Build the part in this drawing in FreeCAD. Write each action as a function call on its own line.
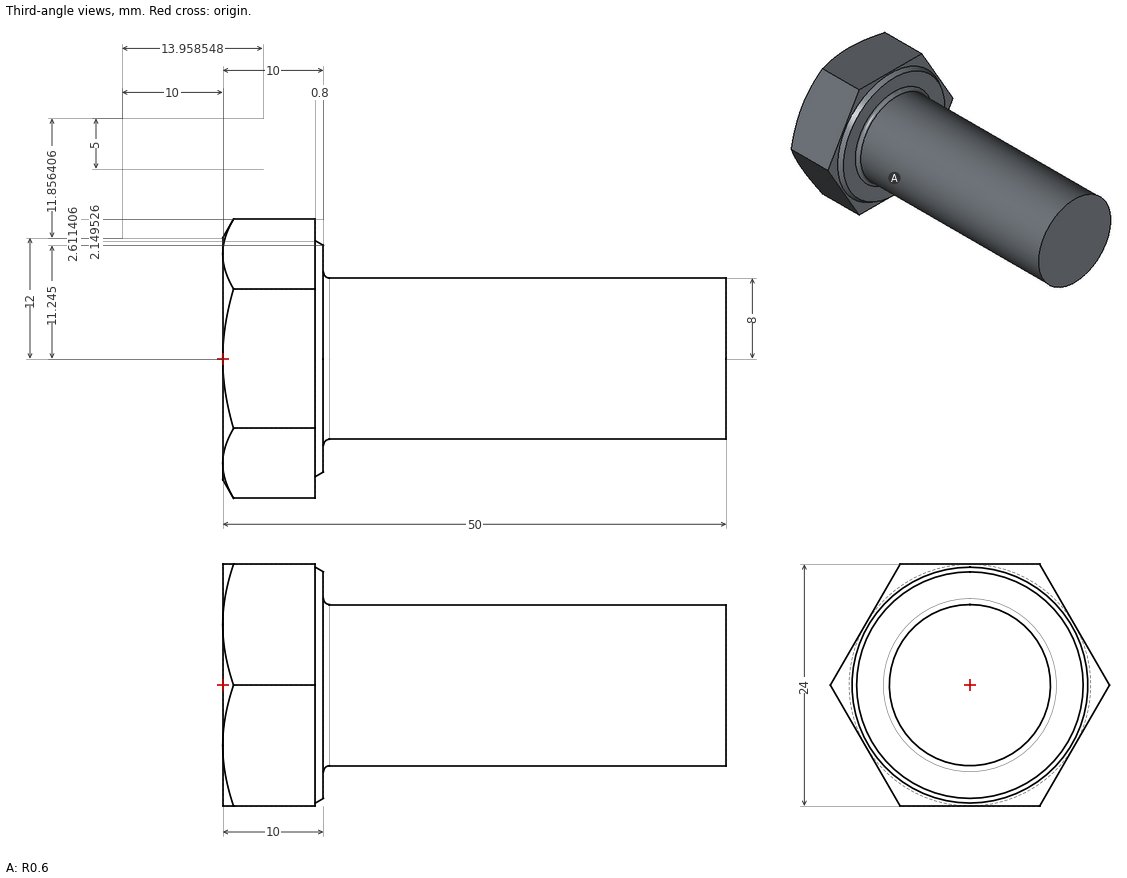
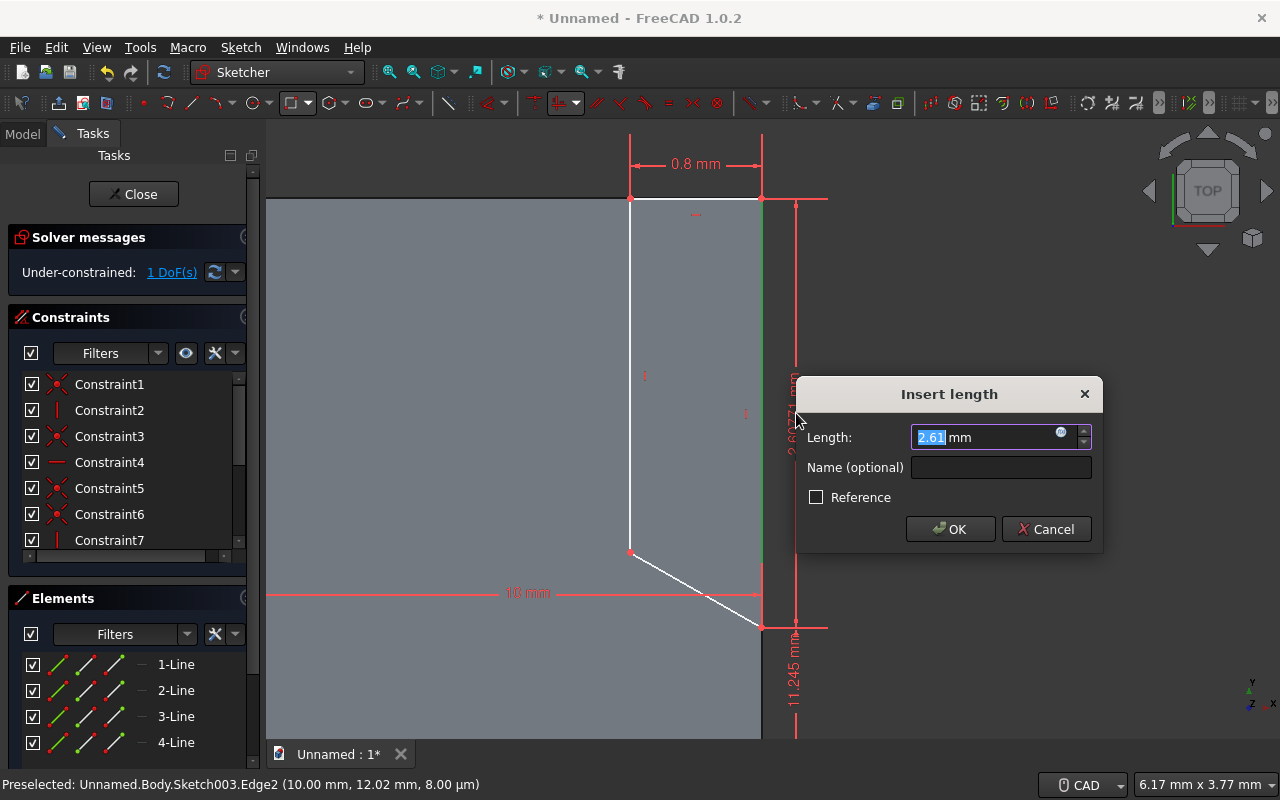
text(2.611406)
key(Return)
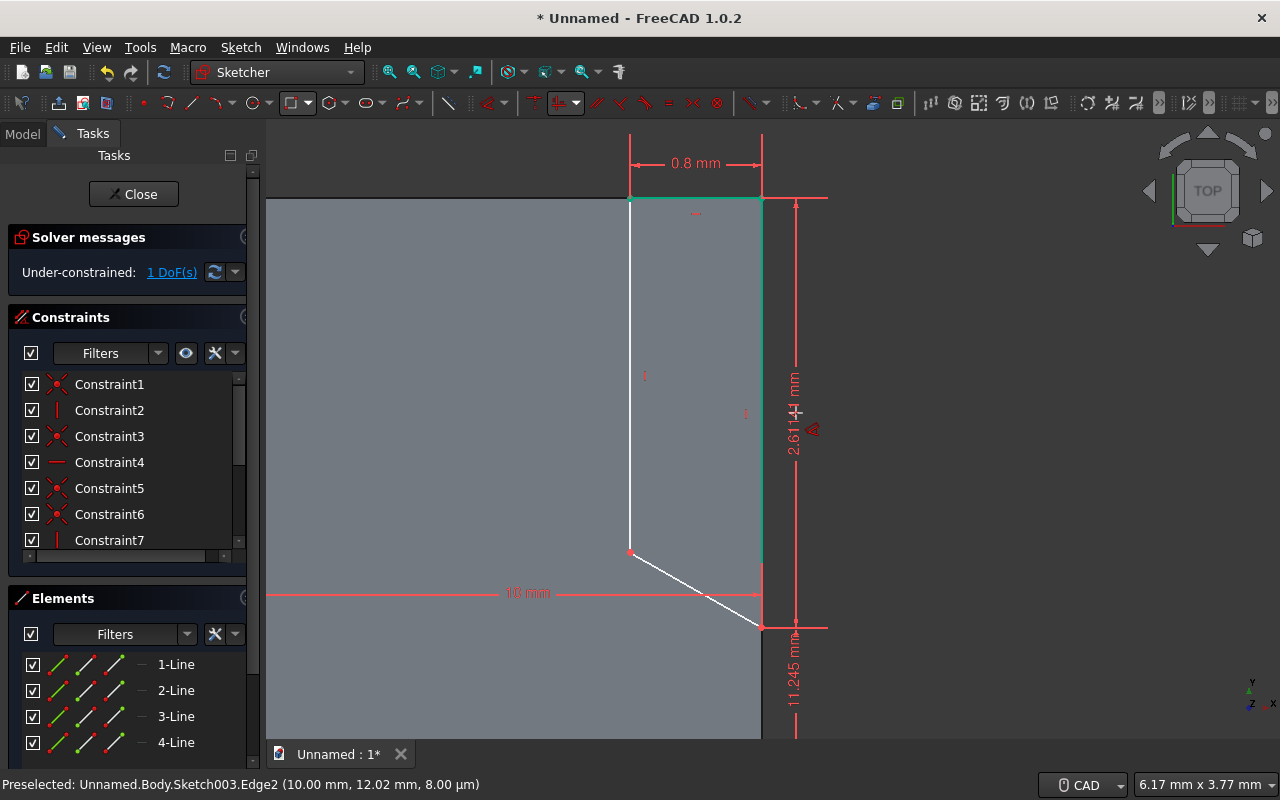
click(630, 305)
click(596, 376)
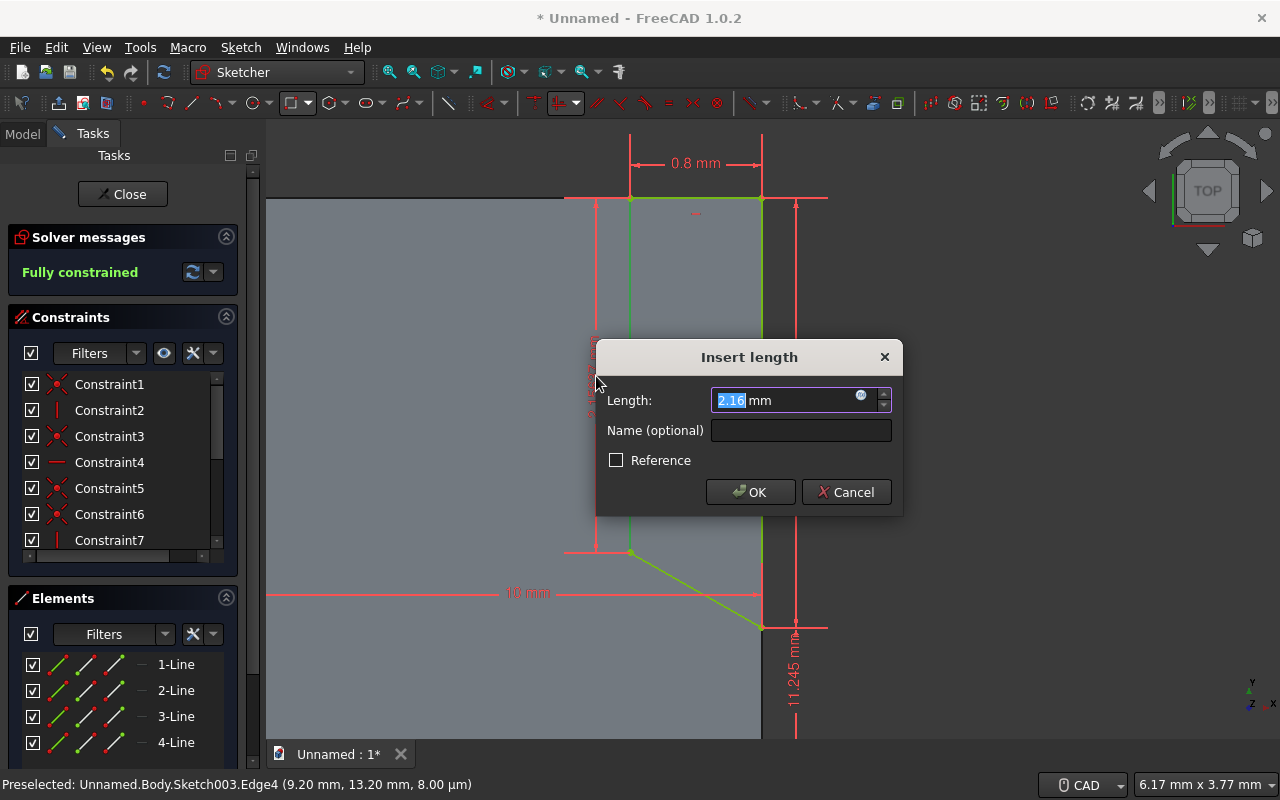
text(2.149526)
key(Return)
key(Escape)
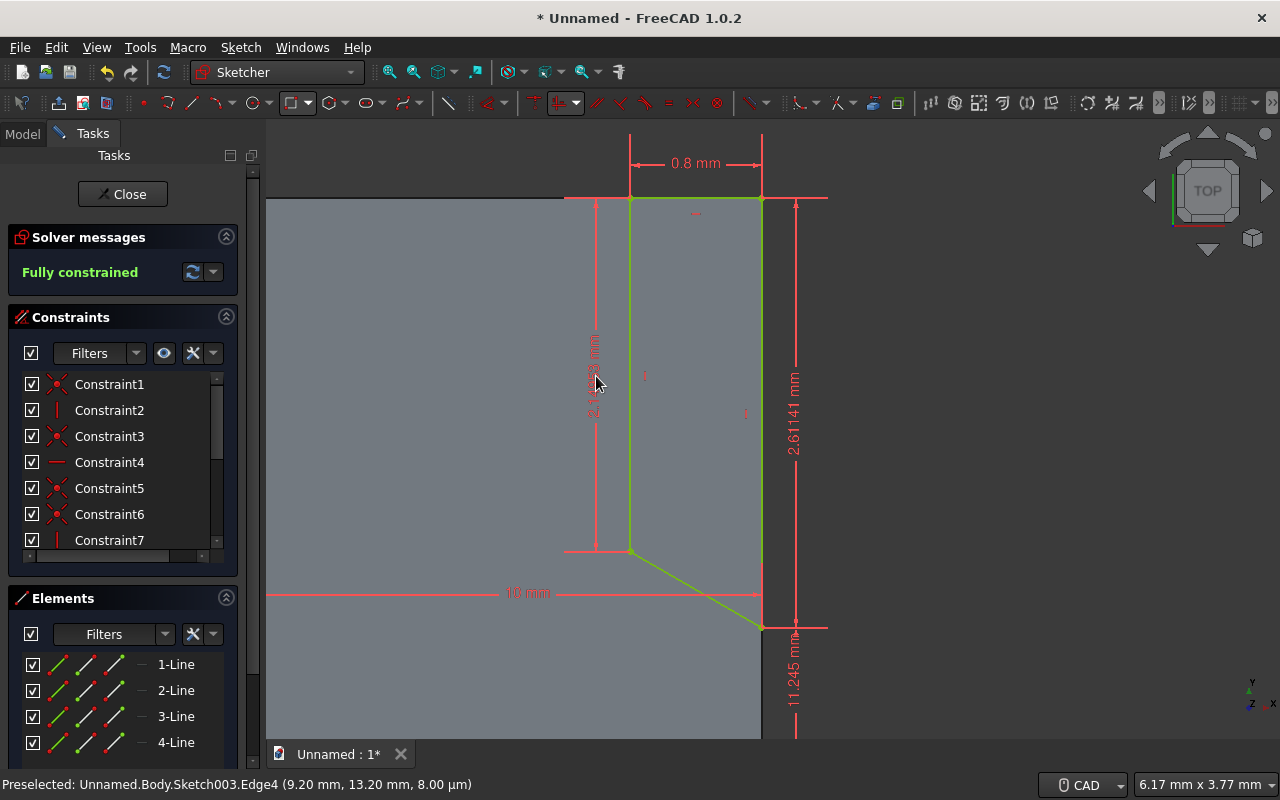
click(123, 194)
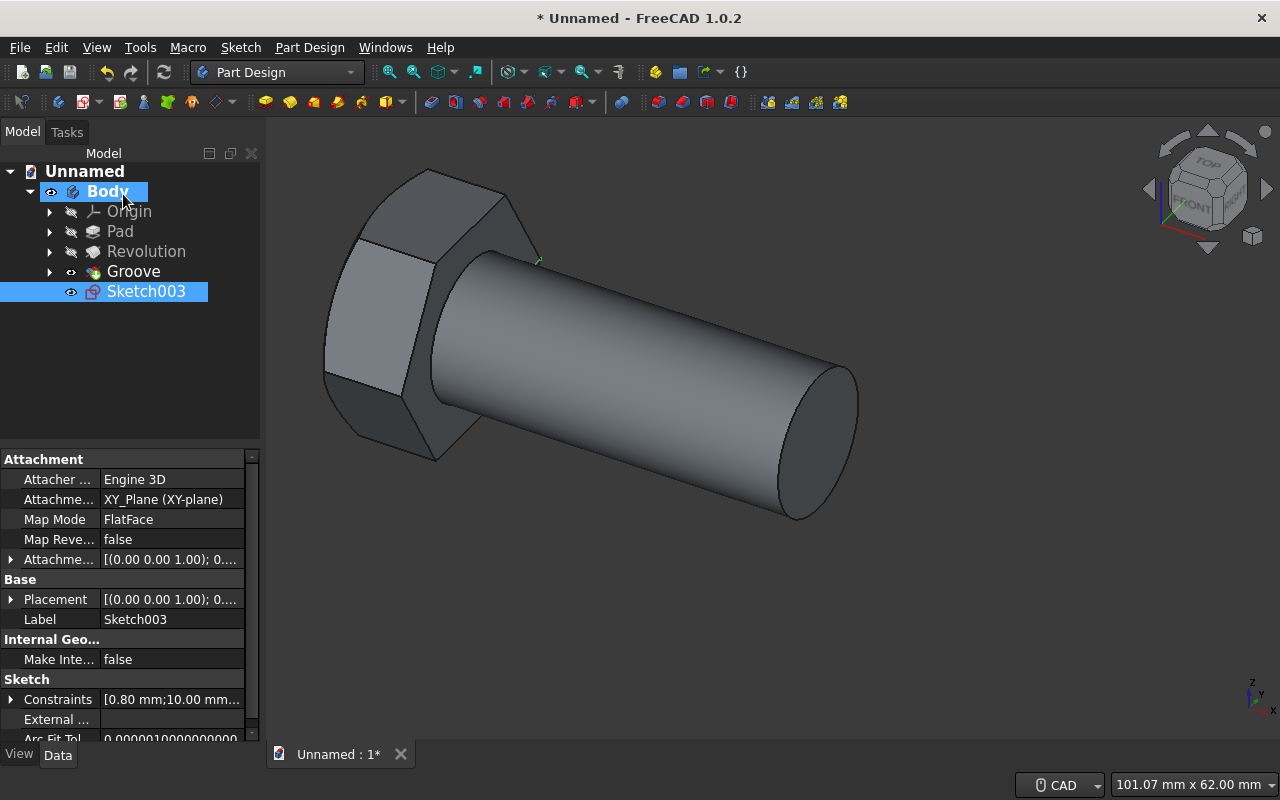
click(480, 102)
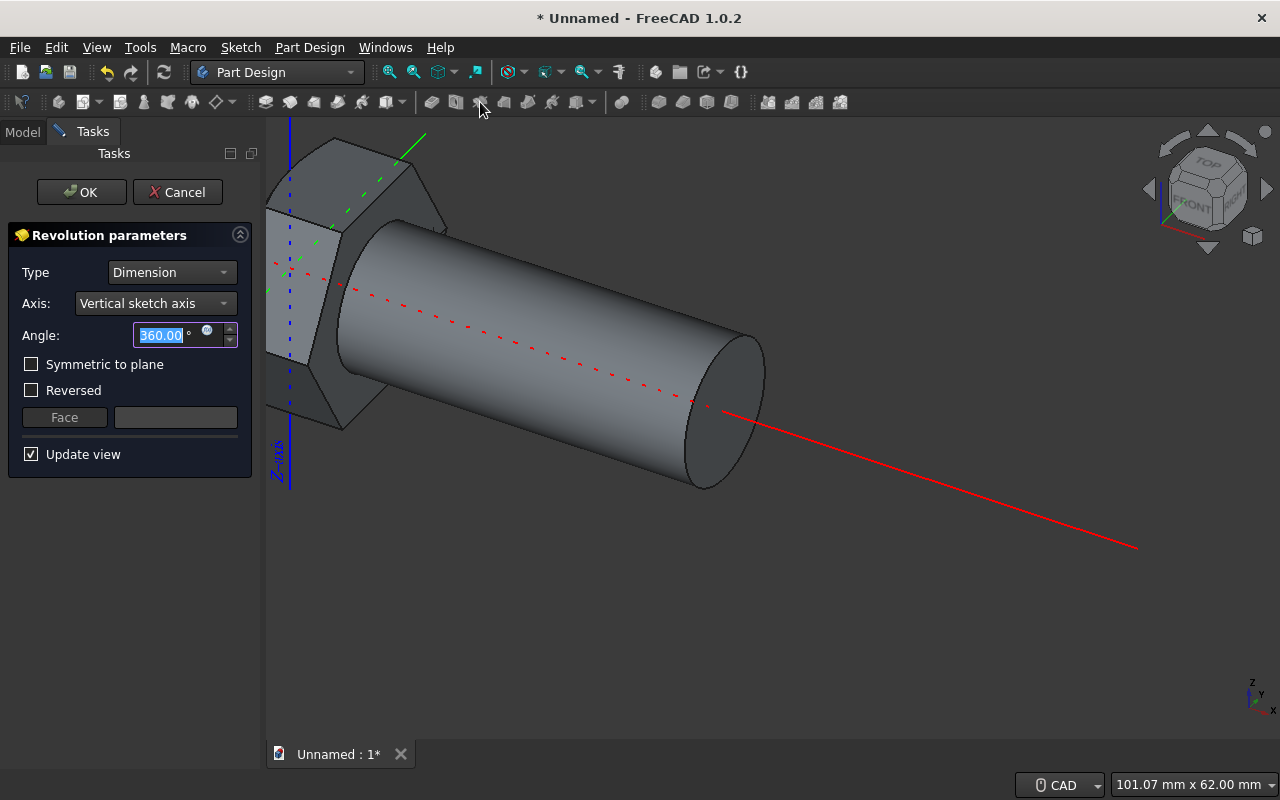
click(156, 304)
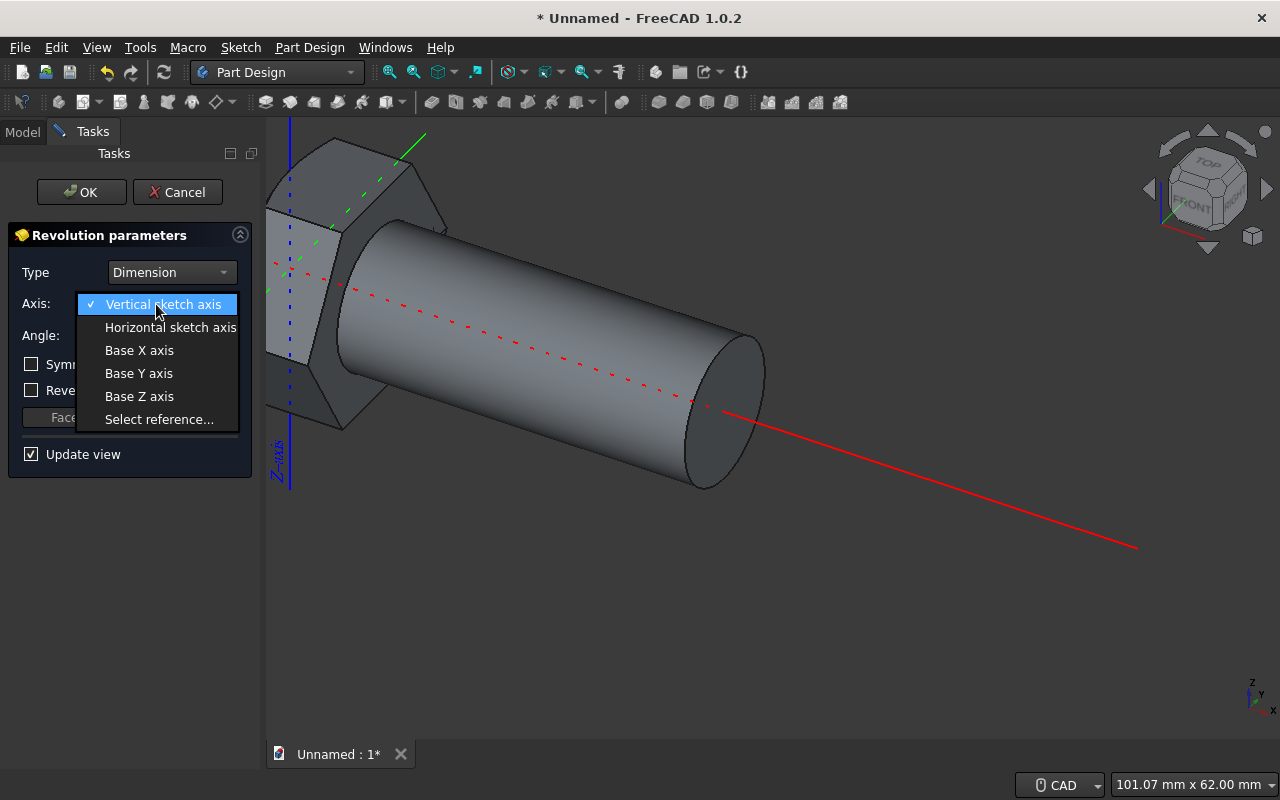
click(156, 328)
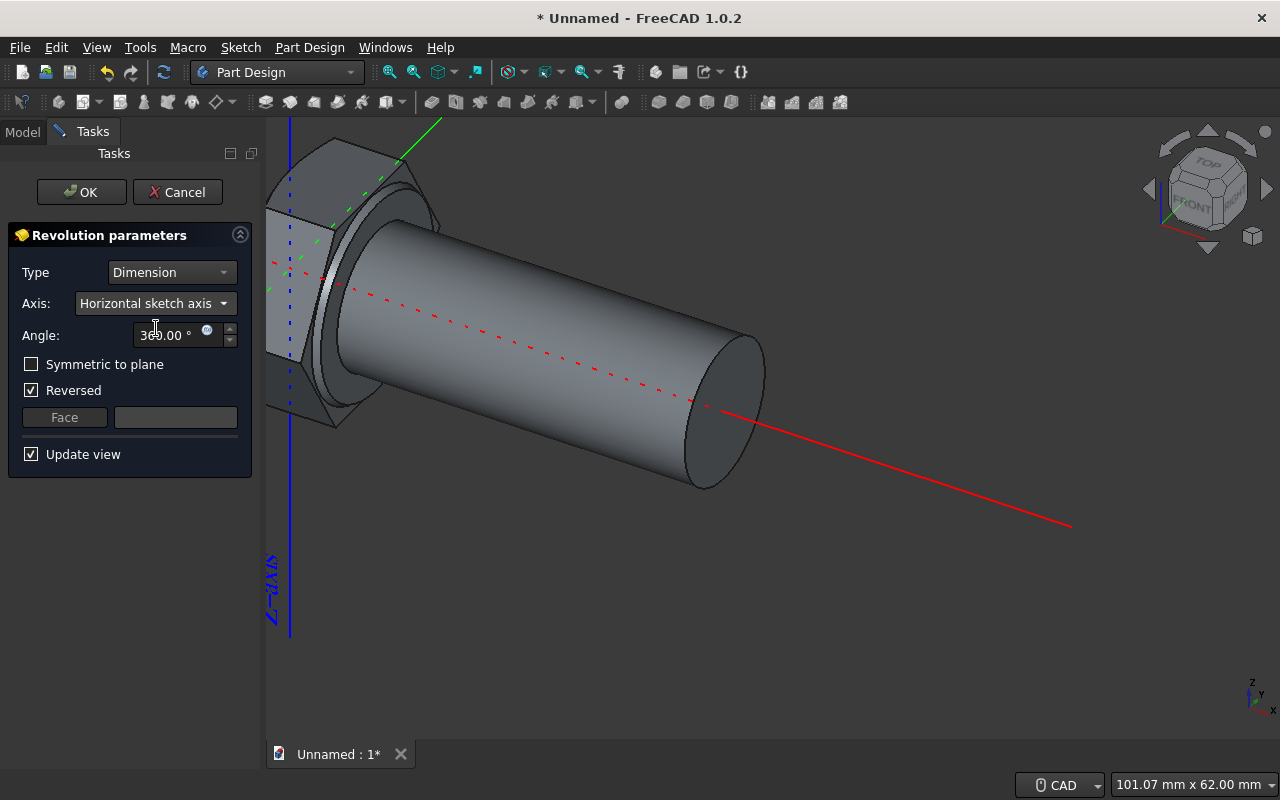
click(82, 192)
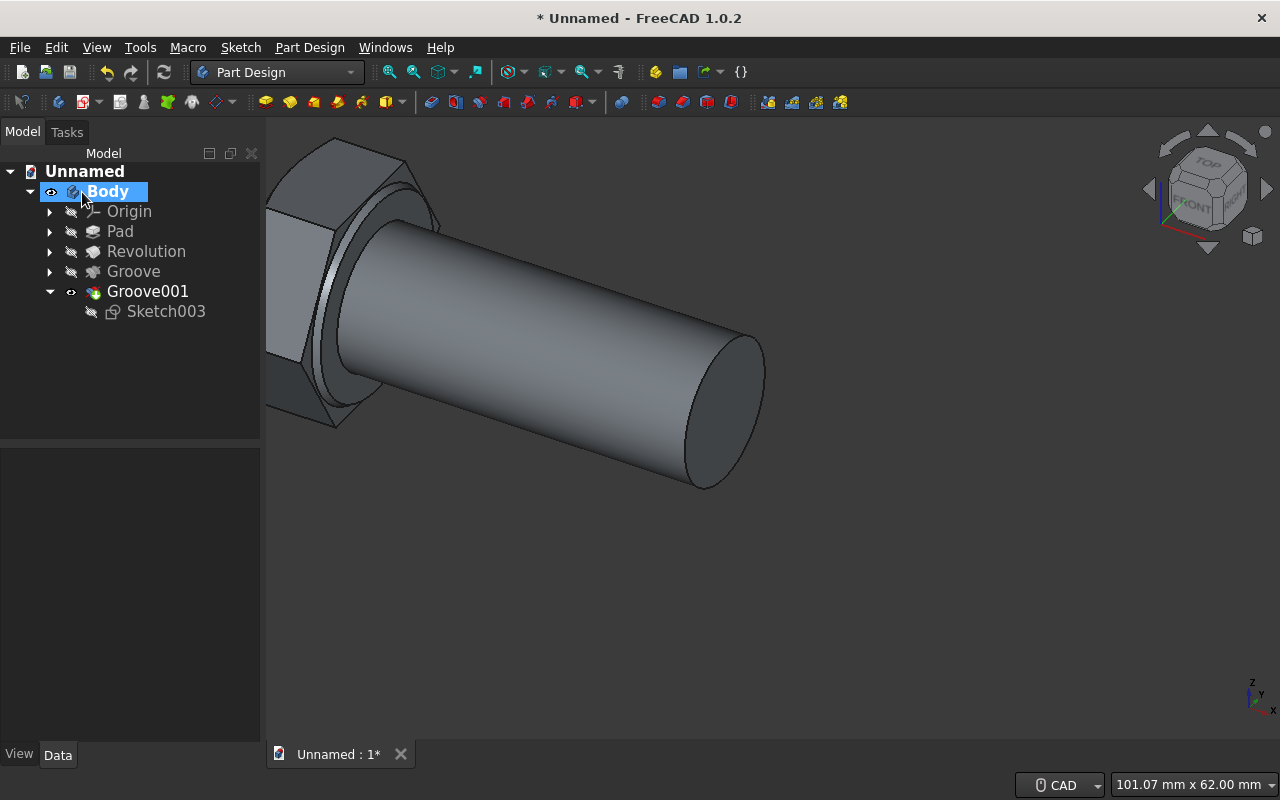
click(390, 72)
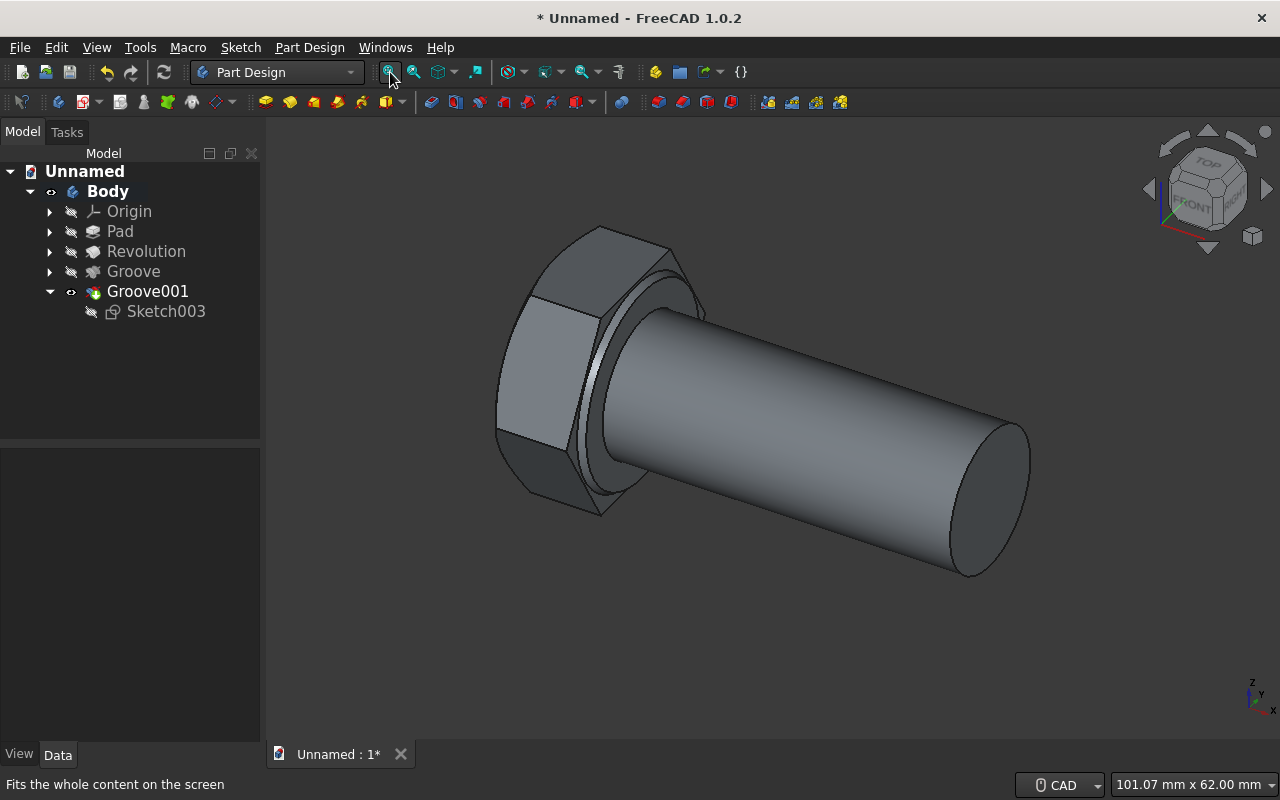
key(0)